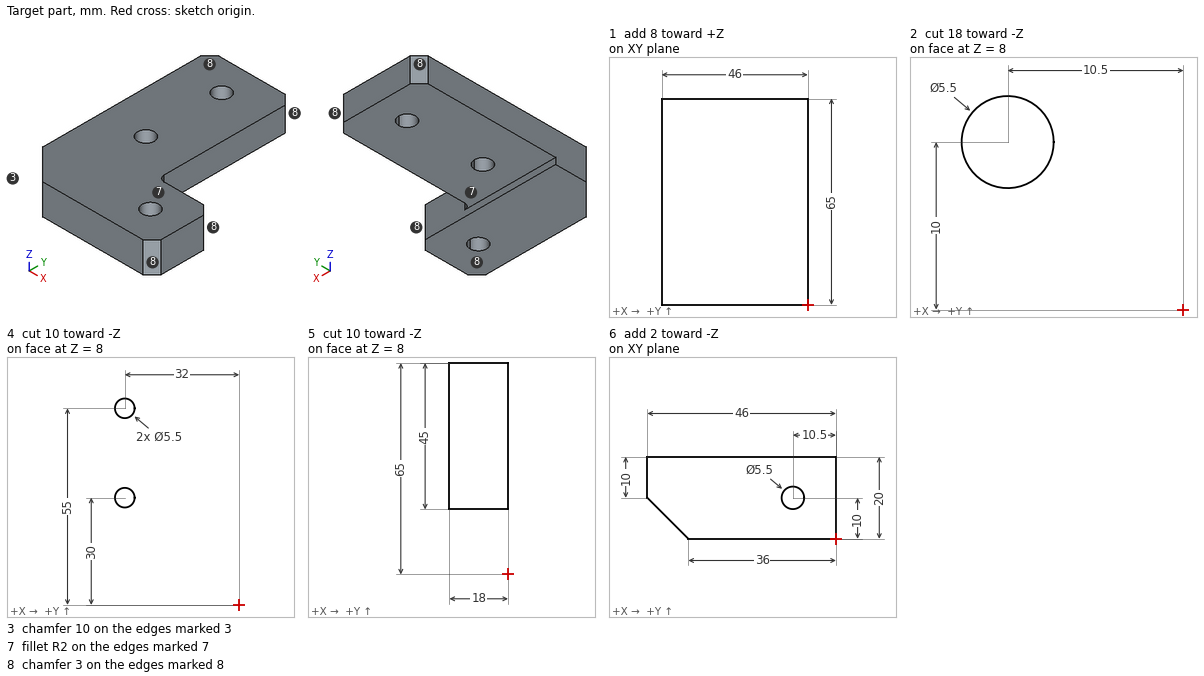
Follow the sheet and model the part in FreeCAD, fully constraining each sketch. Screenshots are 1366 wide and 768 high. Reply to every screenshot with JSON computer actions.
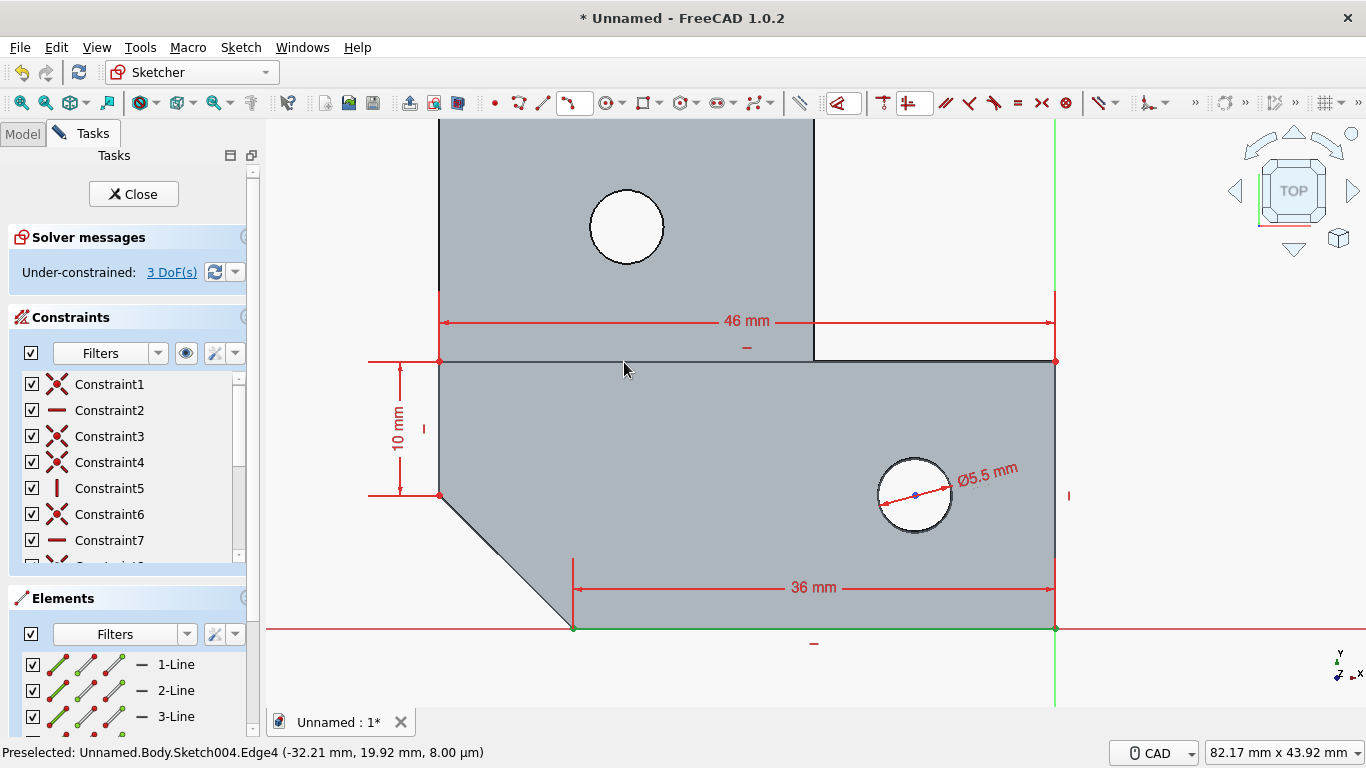
{"action": "left_click", "coordinate": [1055, 442]}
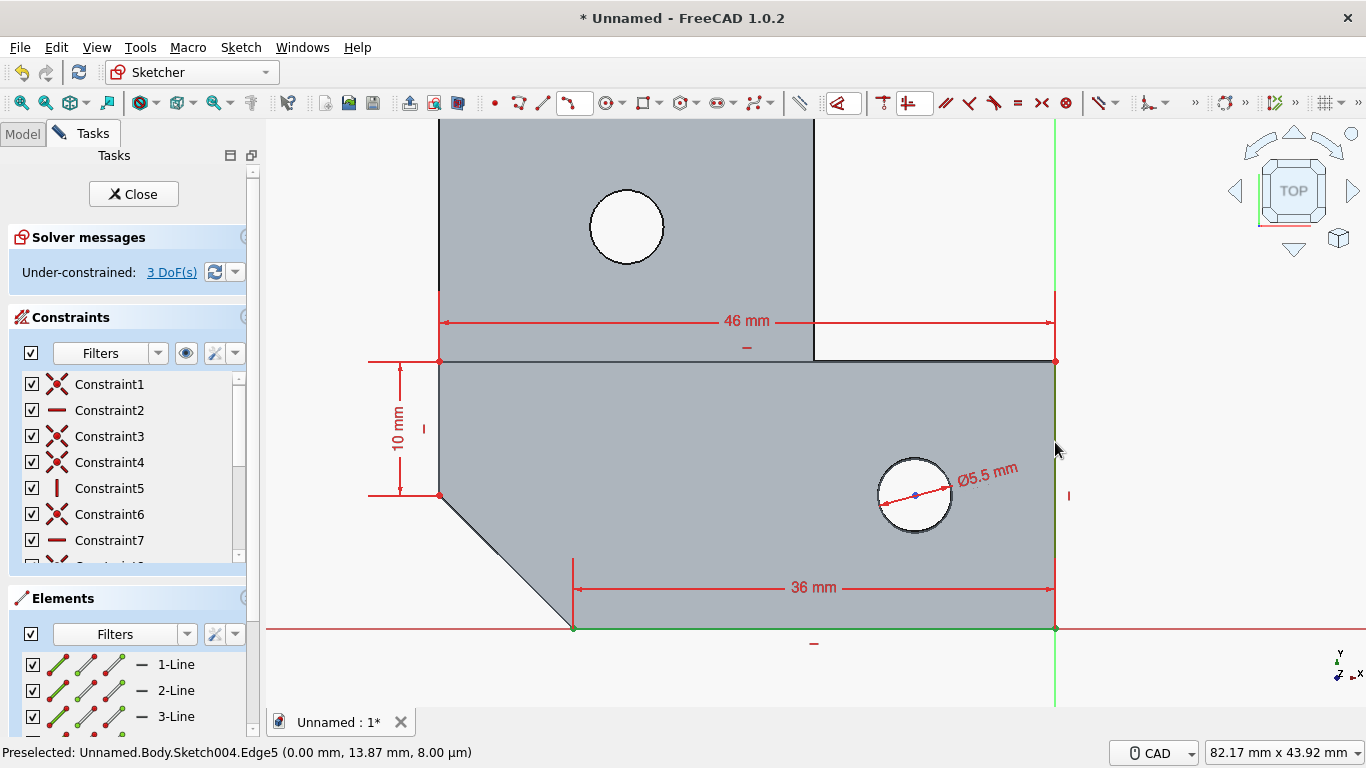
{"action": "left_click", "coordinate": [856, 104]}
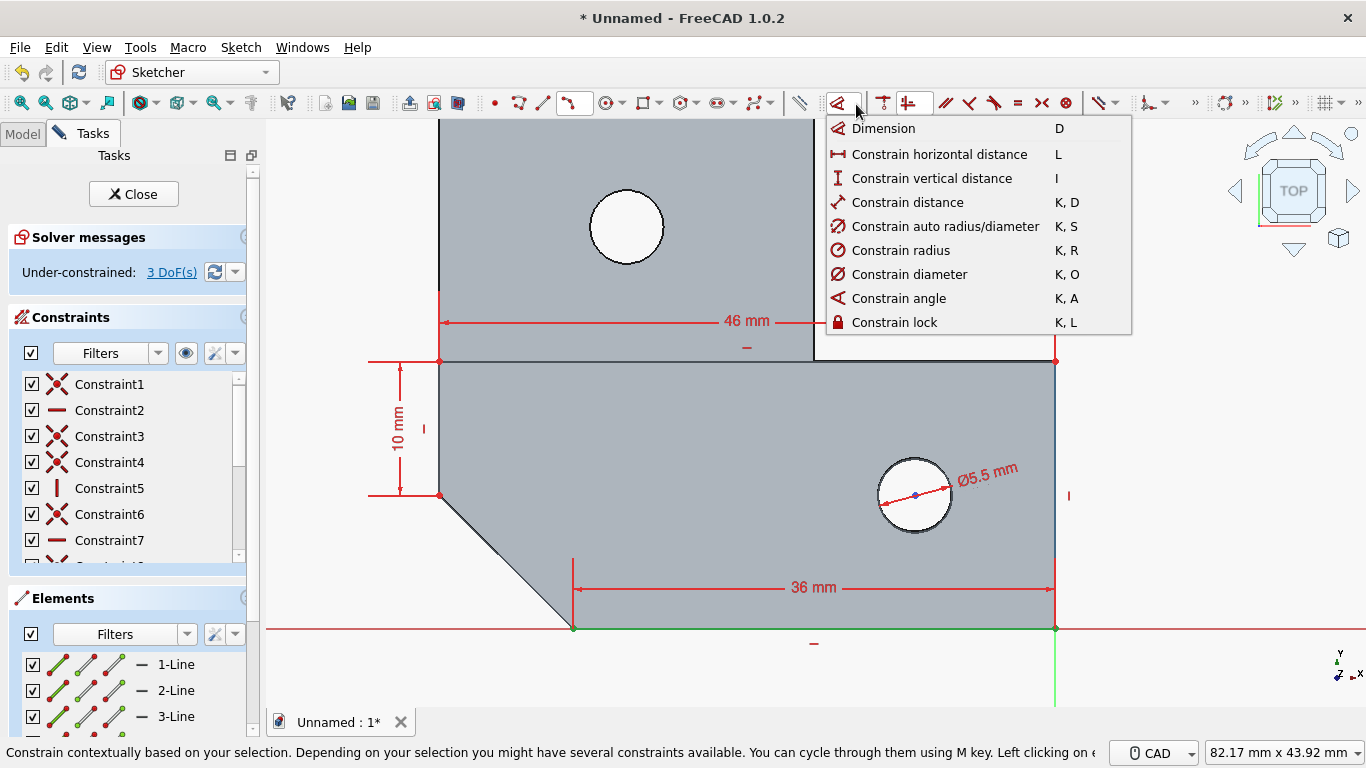
{"action": "left_click", "coordinate": [979, 178]}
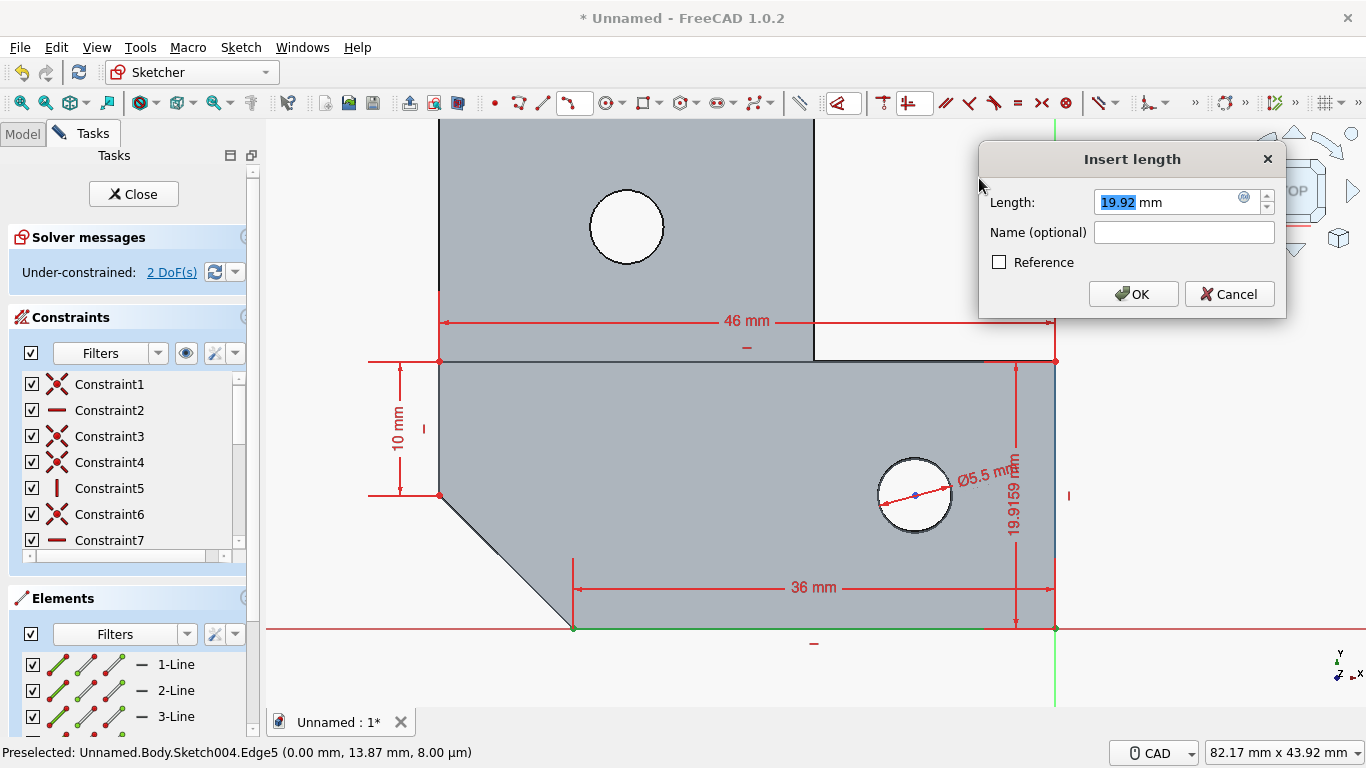
{"action": "type", "text": "20"}
{"action": "key", "text": "Return"}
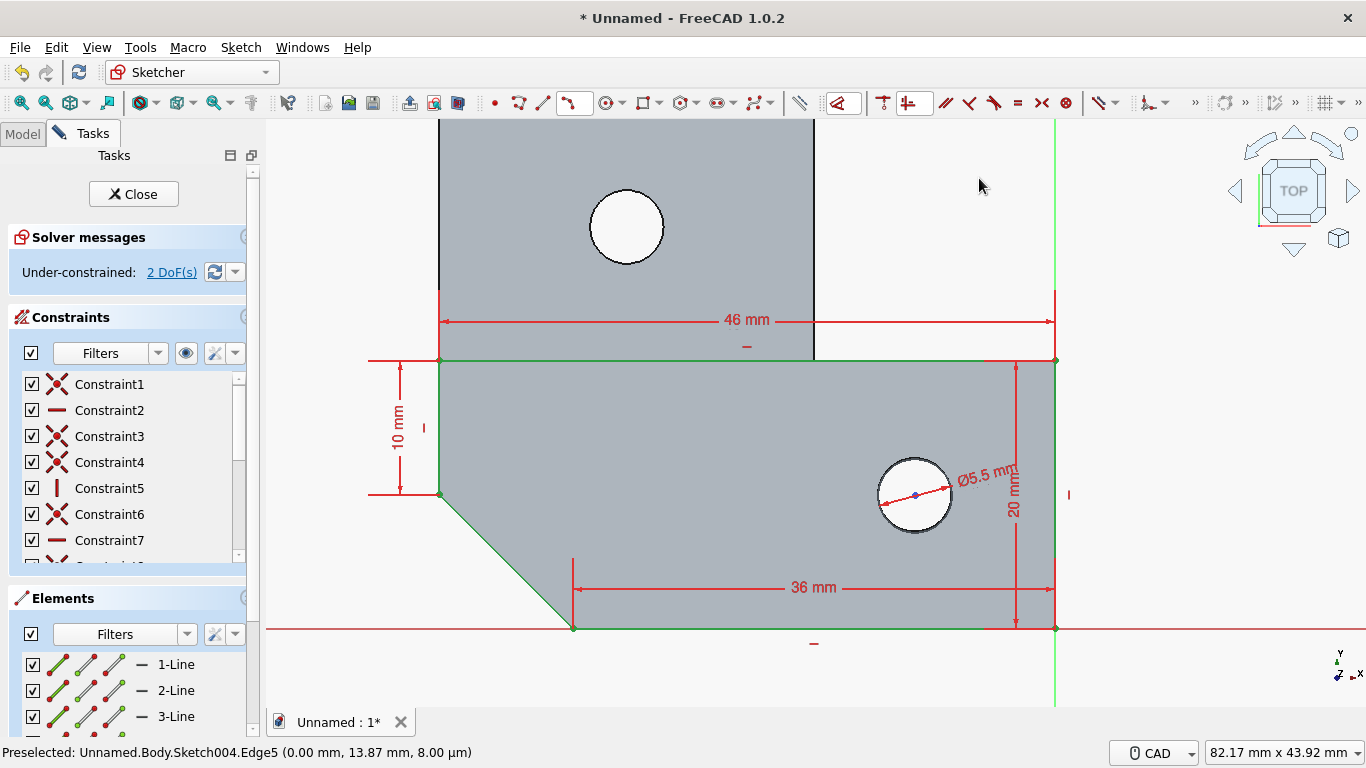
{"action": "left_click", "coordinate": [915, 496]}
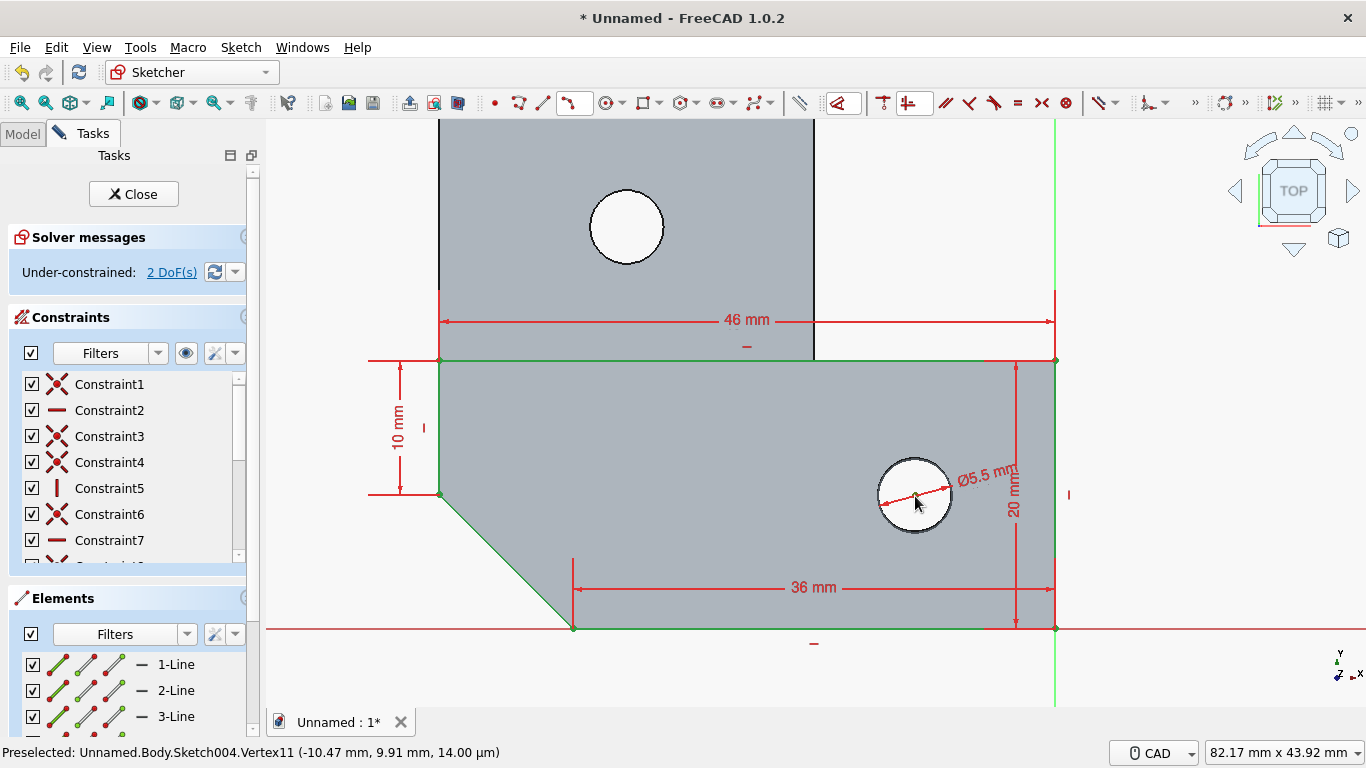
{"action": "key", "text": "i"}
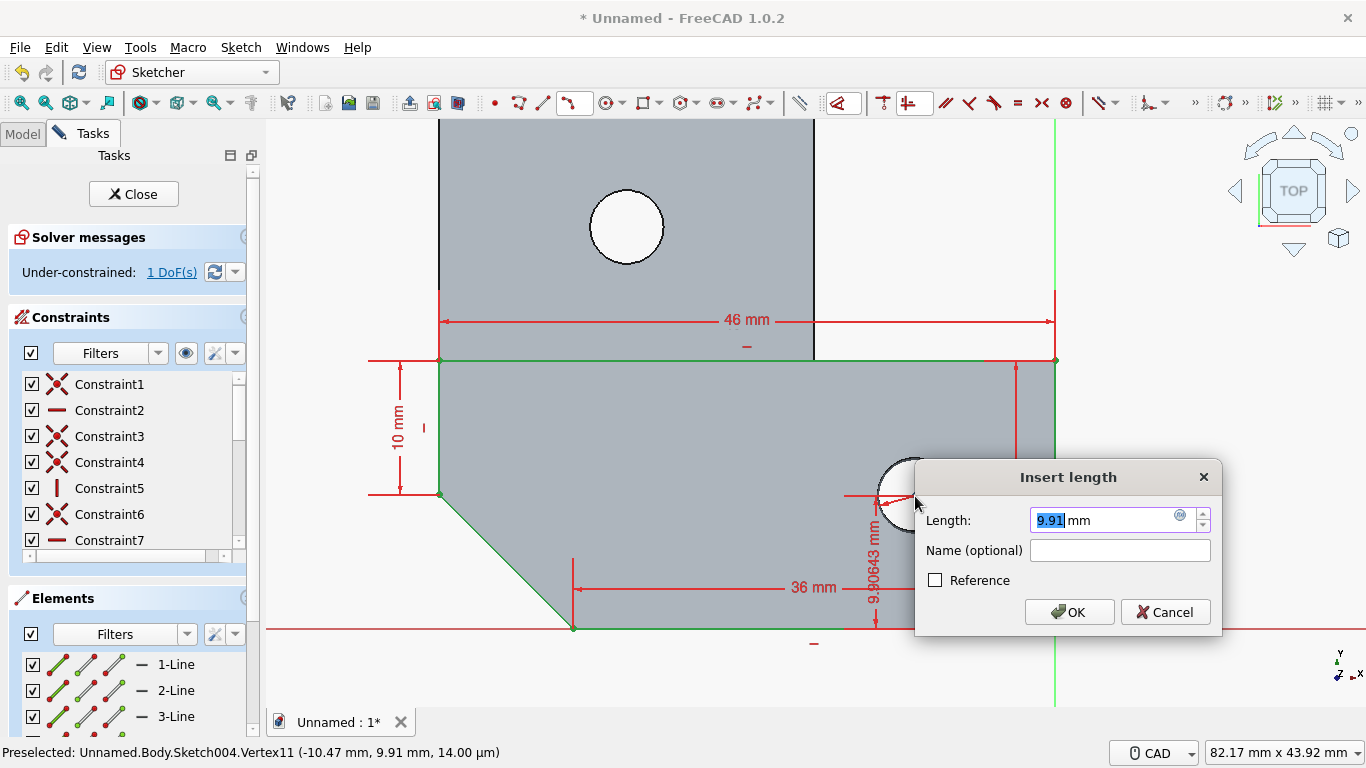
{"action": "type", "text": "10"}
{"action": "key", "text": "Return"}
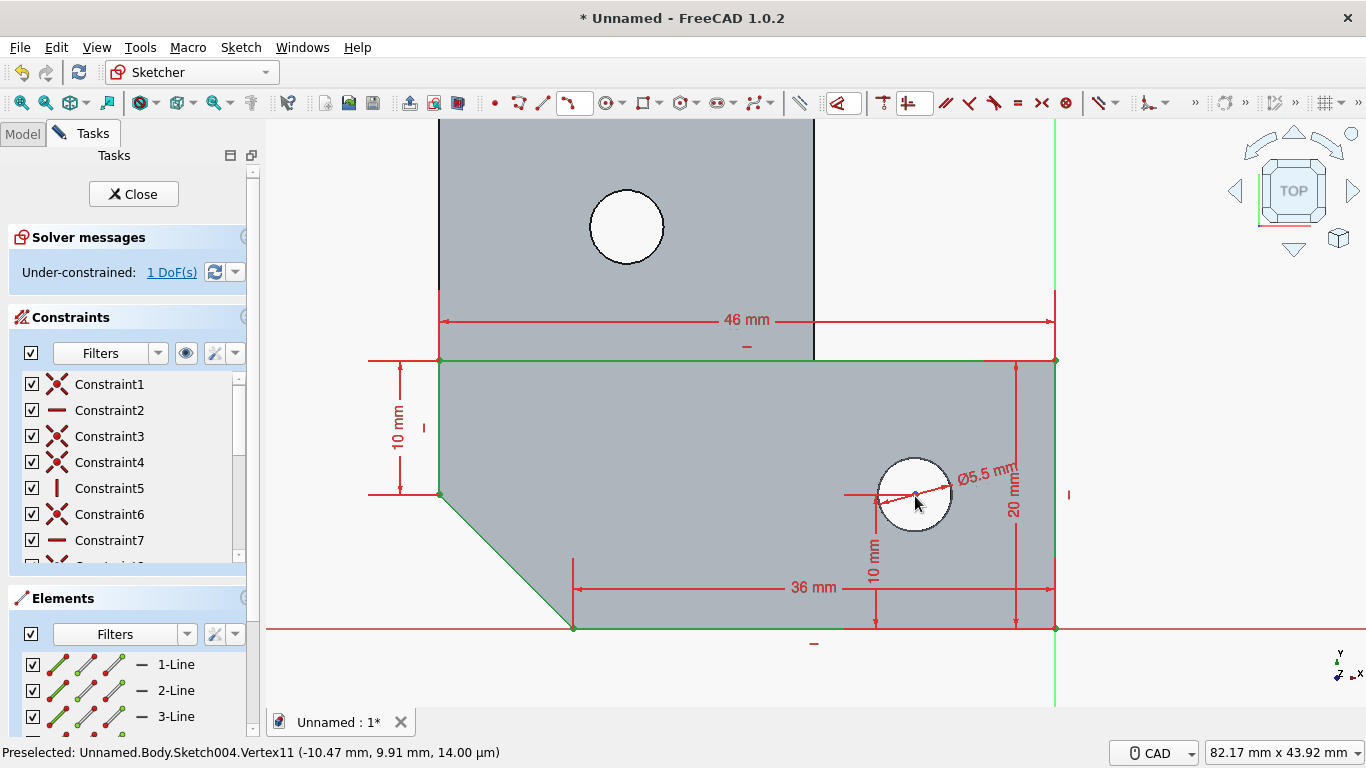
{"action": "left_click", "coordinate": [915, 495]}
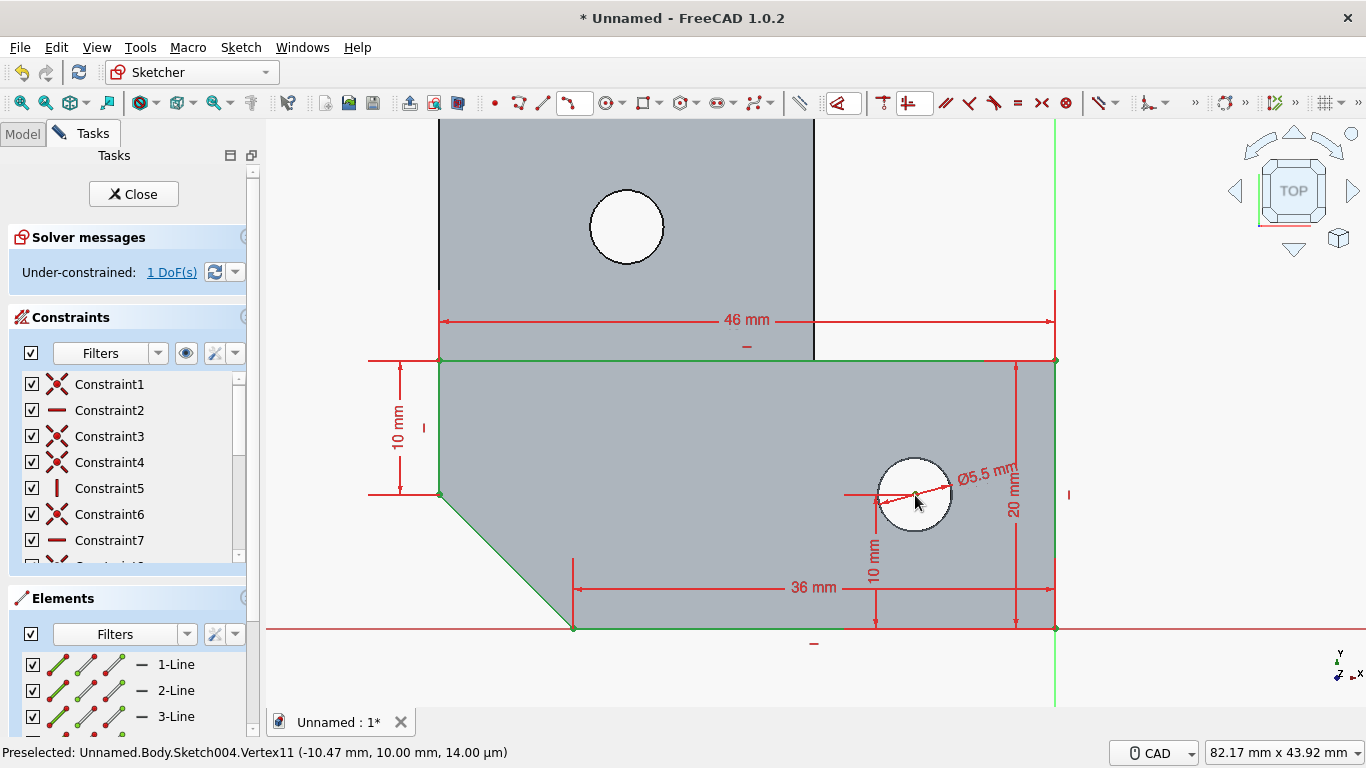
{"action": "left_click", "coordinate": [856, 104]}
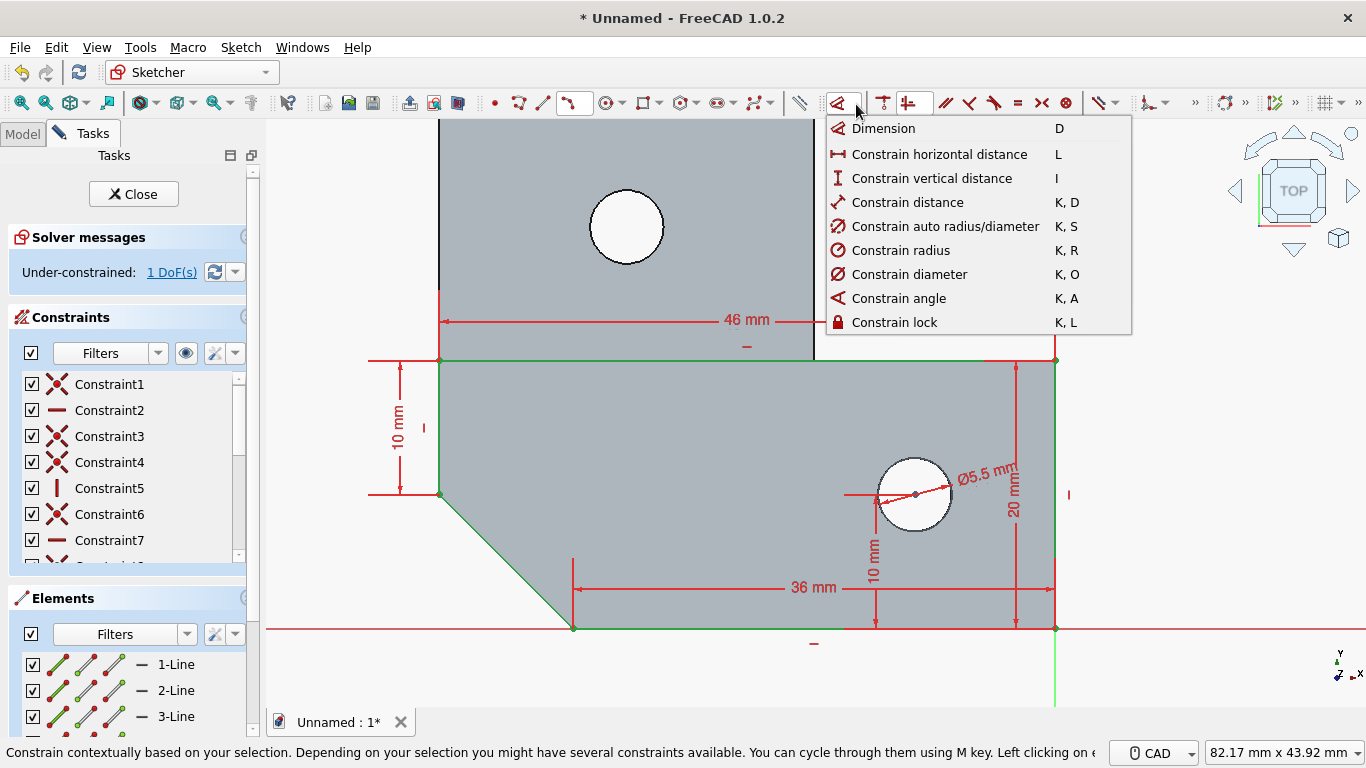
{"action": "left_click", "coordinate": [979, 154]}